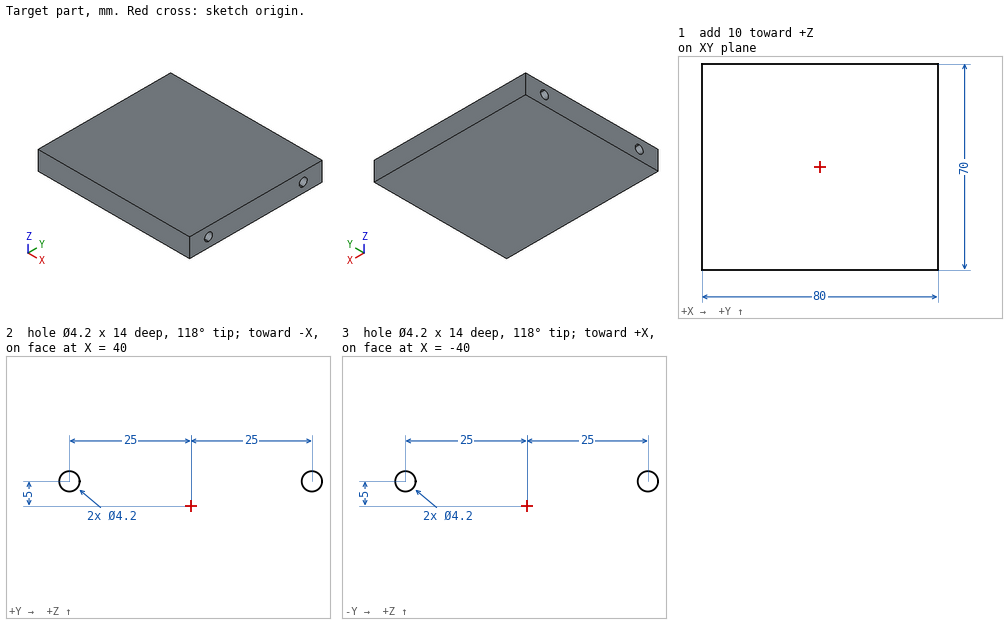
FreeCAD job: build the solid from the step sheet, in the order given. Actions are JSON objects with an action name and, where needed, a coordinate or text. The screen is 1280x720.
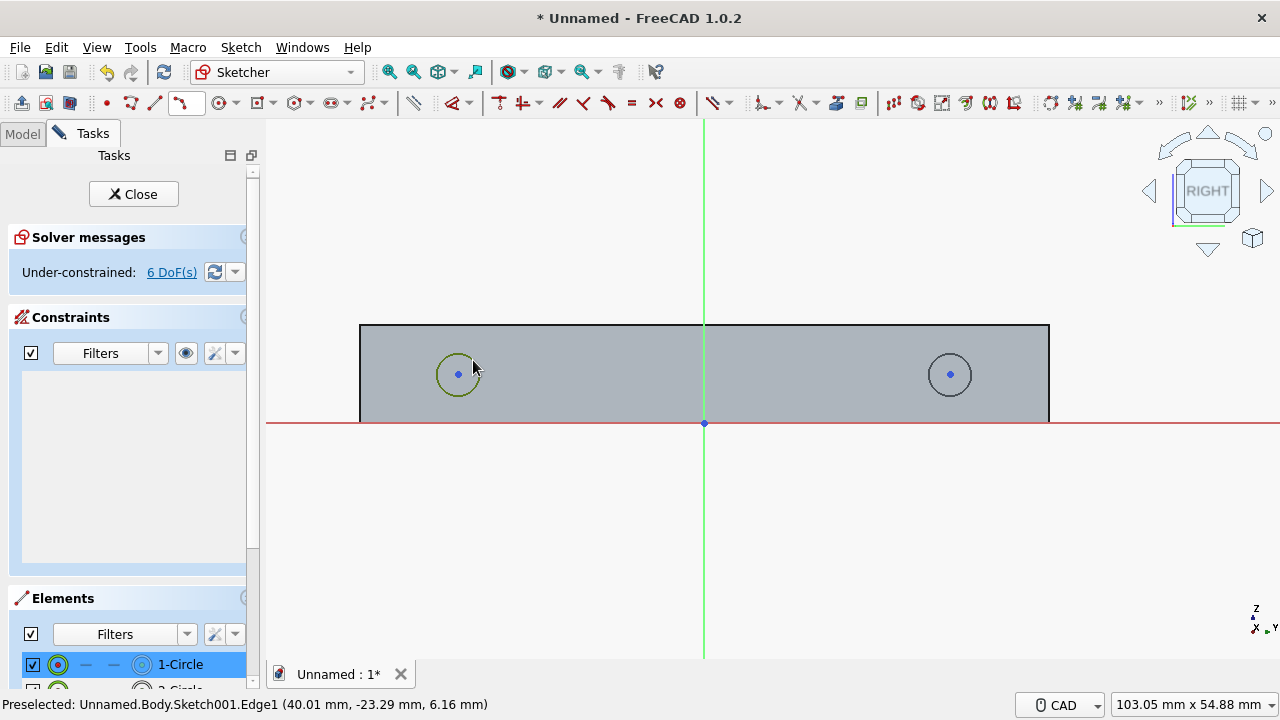
{"action": "left_click", "coordinate": [965, 360]}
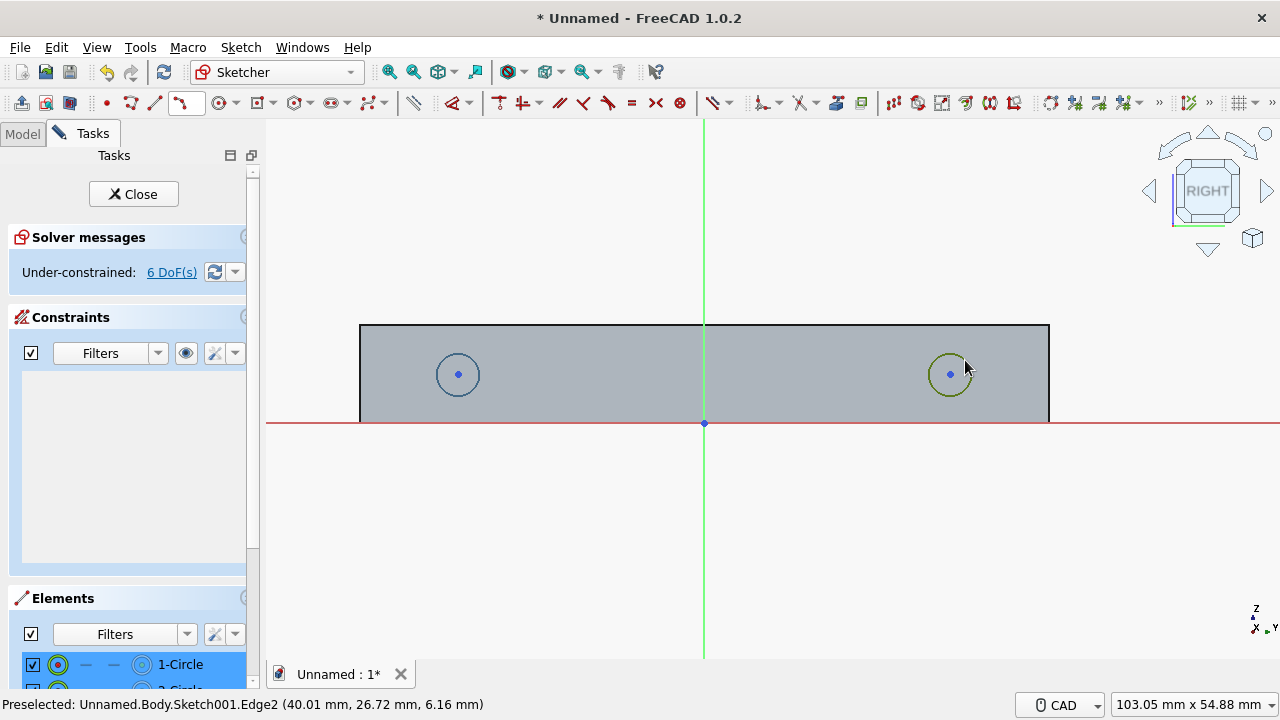
{"action": "left_click", "coordinate": [632, 104]}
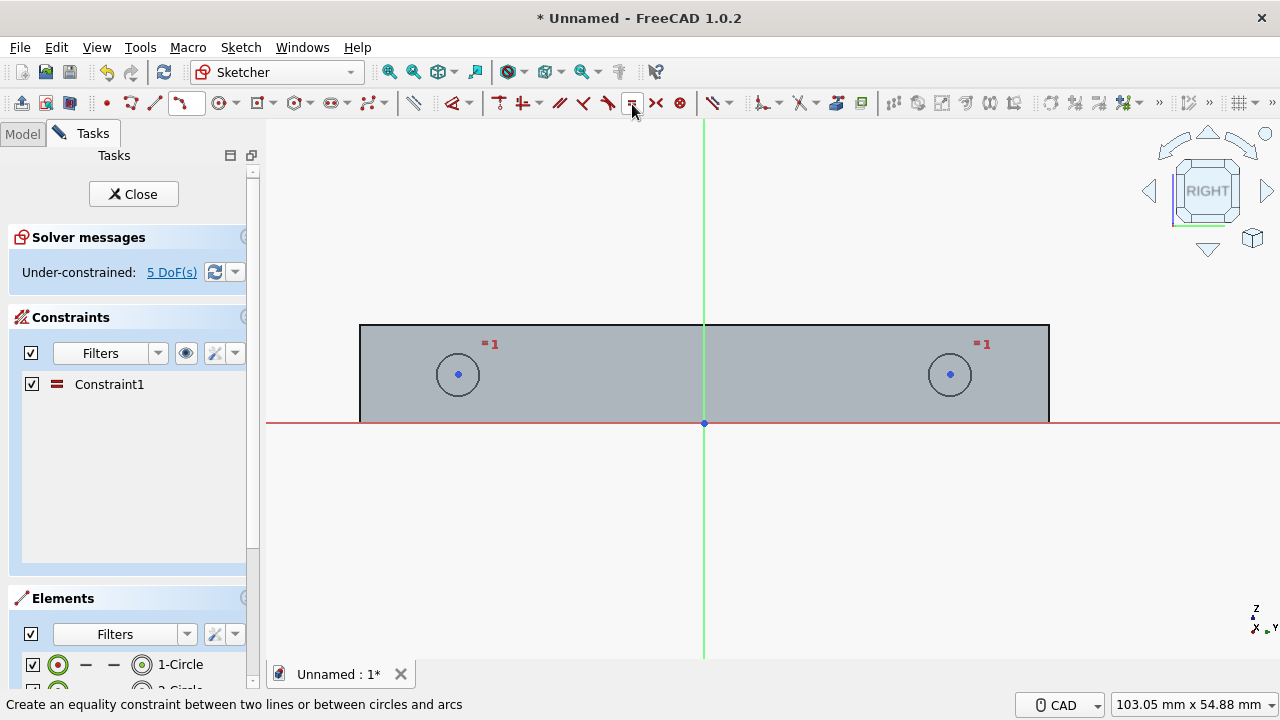
{"action": "left_click", "coordinate": [458, 375]}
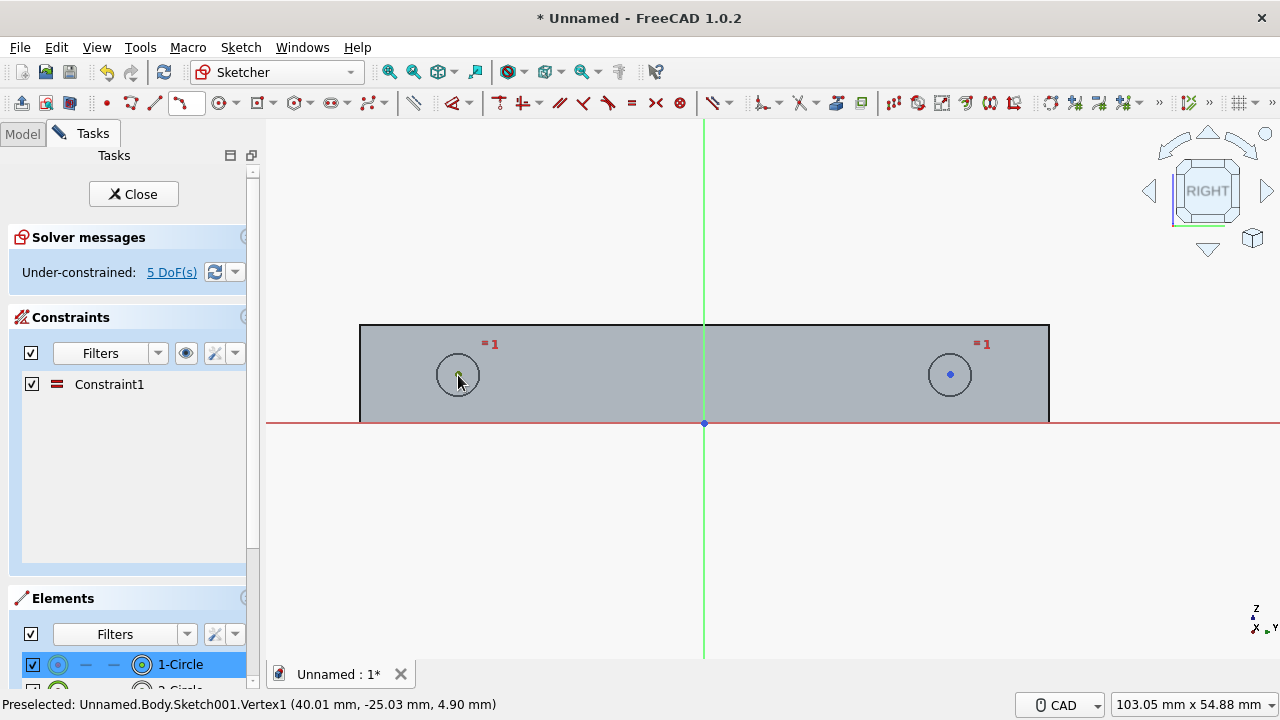
{"action": "left_click", "coordinate": [950, 375]}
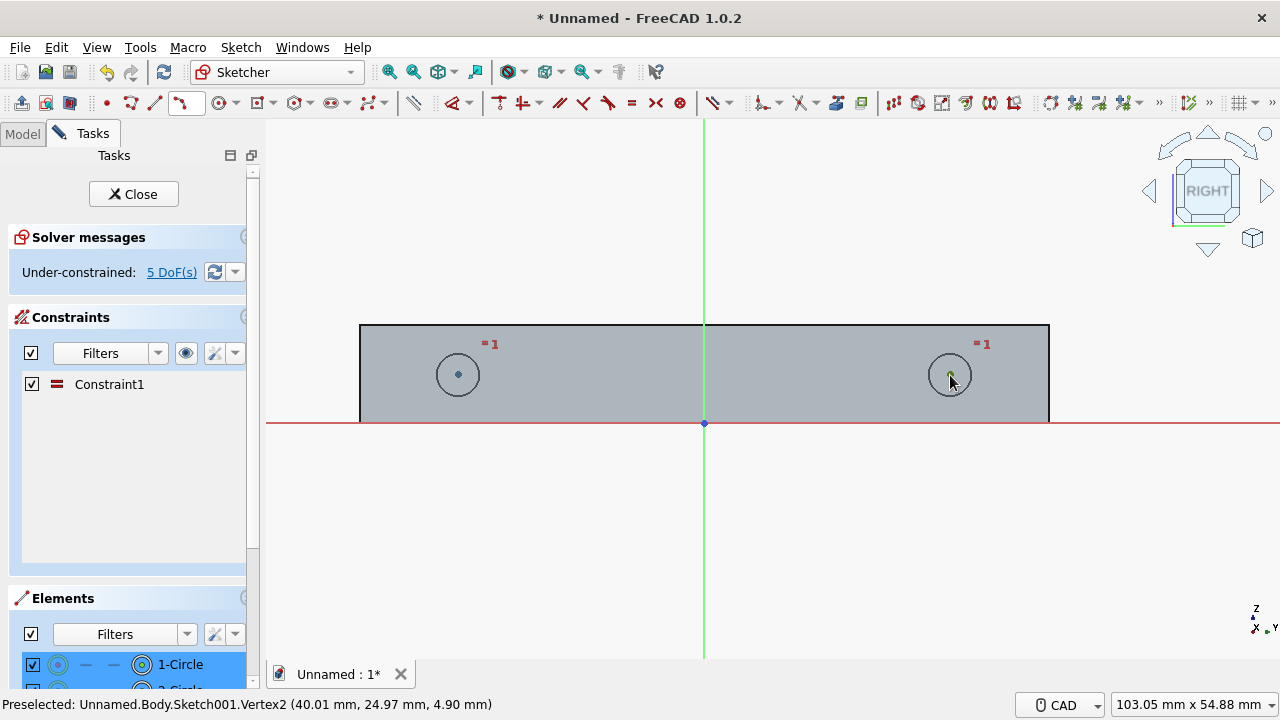
{"action": "key", "text": "h"}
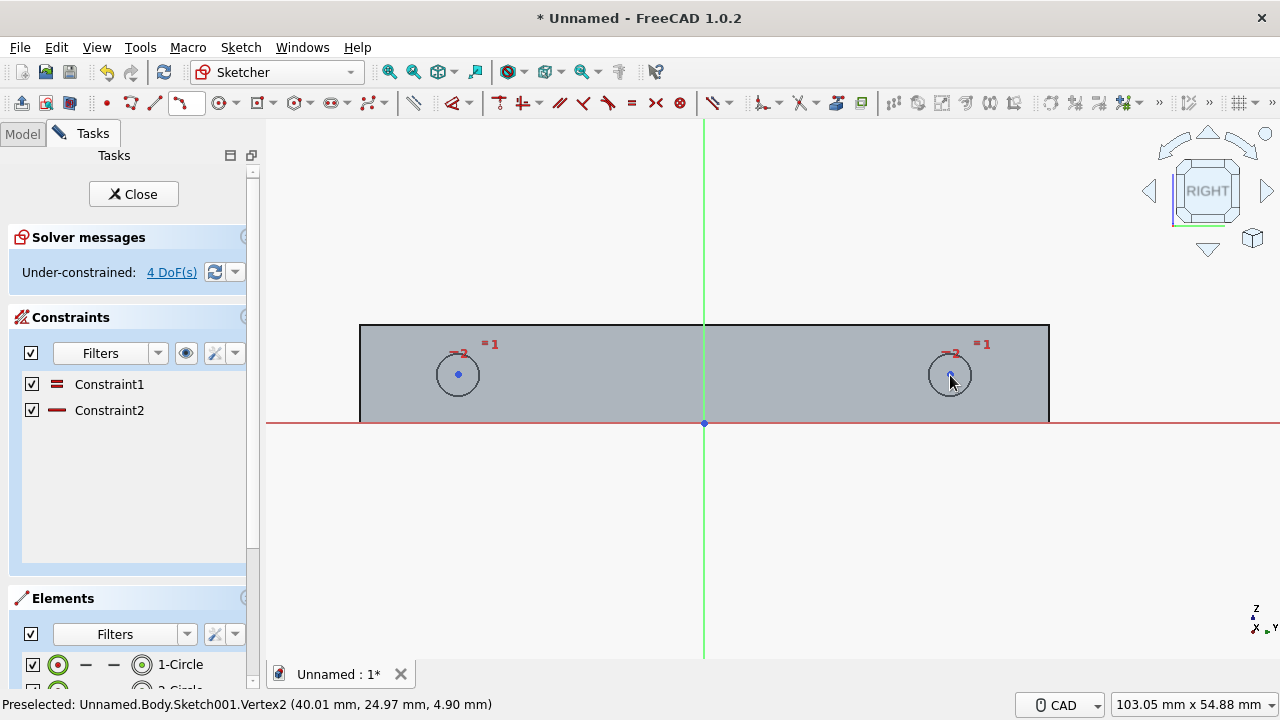
{"action": "left_click", "coordinate": [452, 104]}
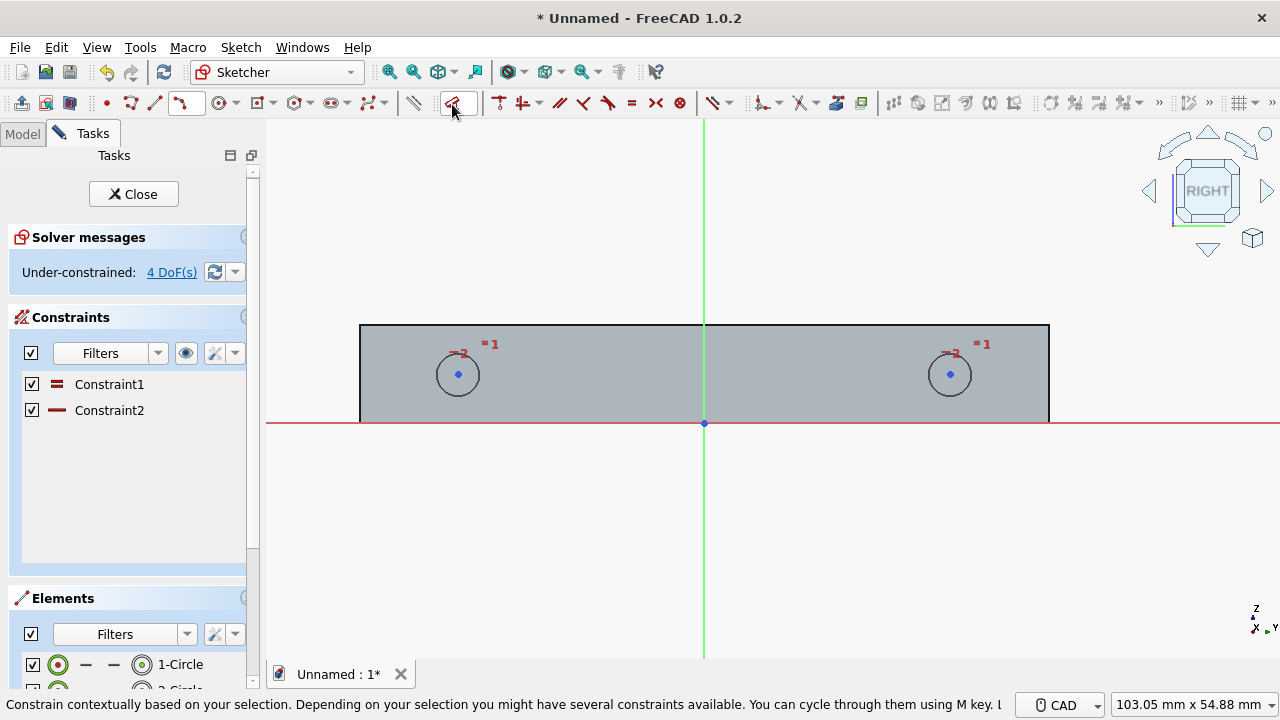
{"action": "left_click", "coordinate": [473, 360]}
{"action": "left_click", "coordinate": [496, 337]}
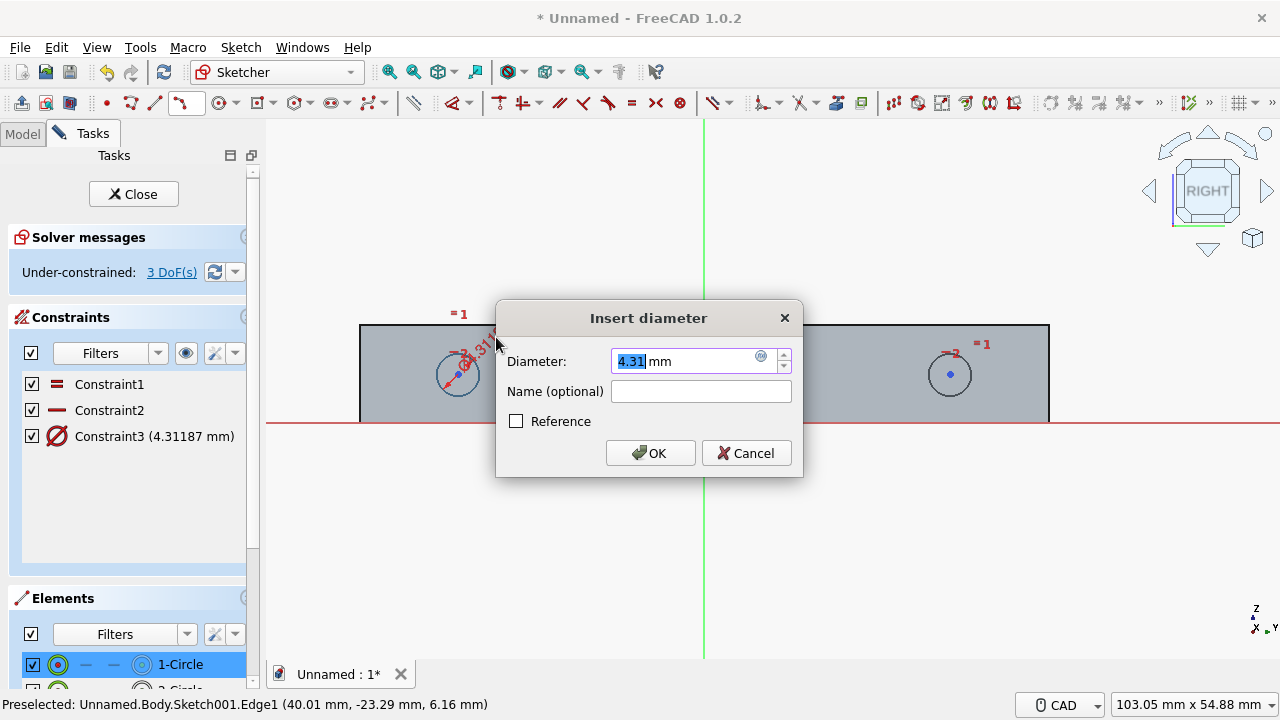
{"action": "type", "text": "4.2"}
{"action": "key", "text": "Return"}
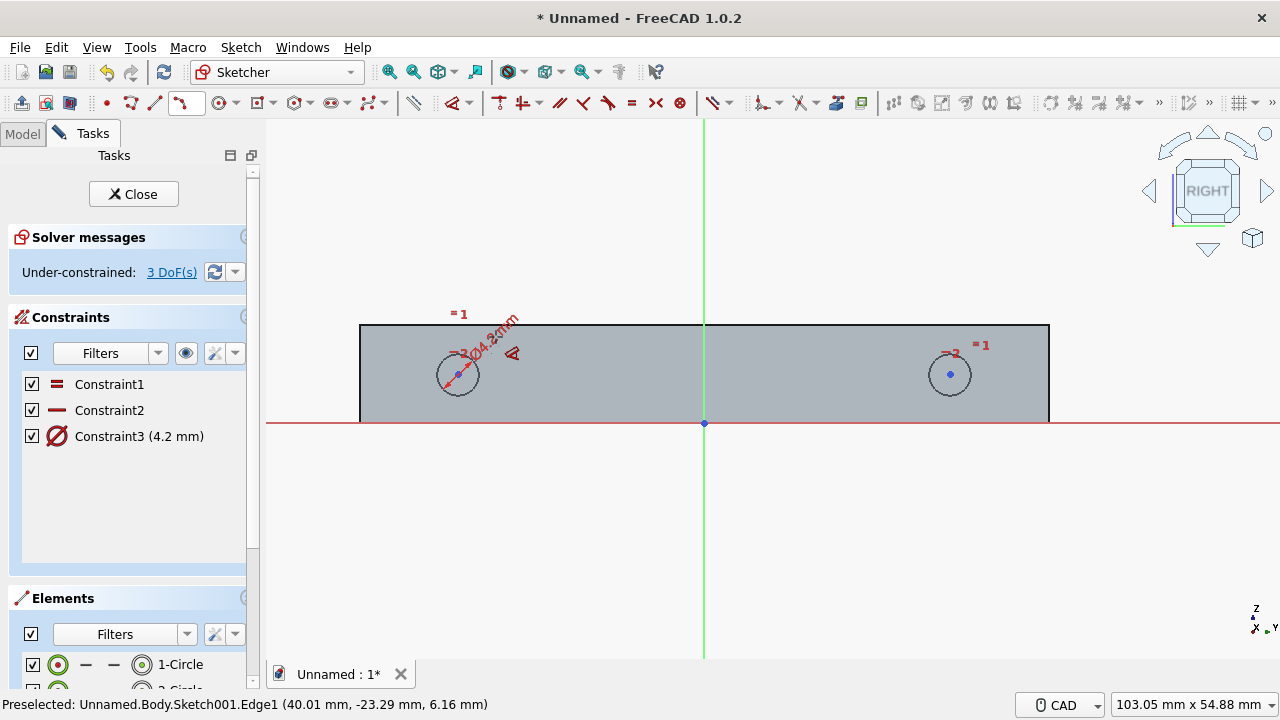
{"action": "left_click", "coordinate": [458, 375]}
{"action": "left_click", "coordinate": [424, 399]}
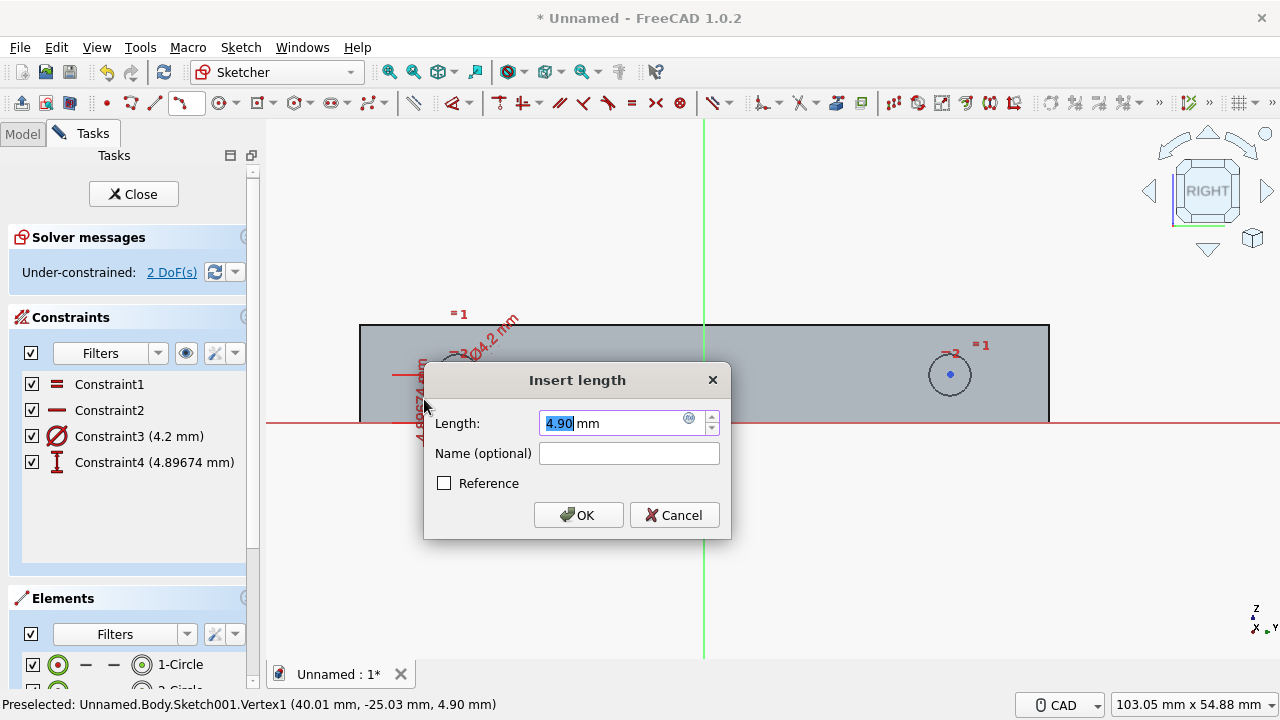
{"action": "type", "text": "5"}
{"action": "key", "text": "Return"}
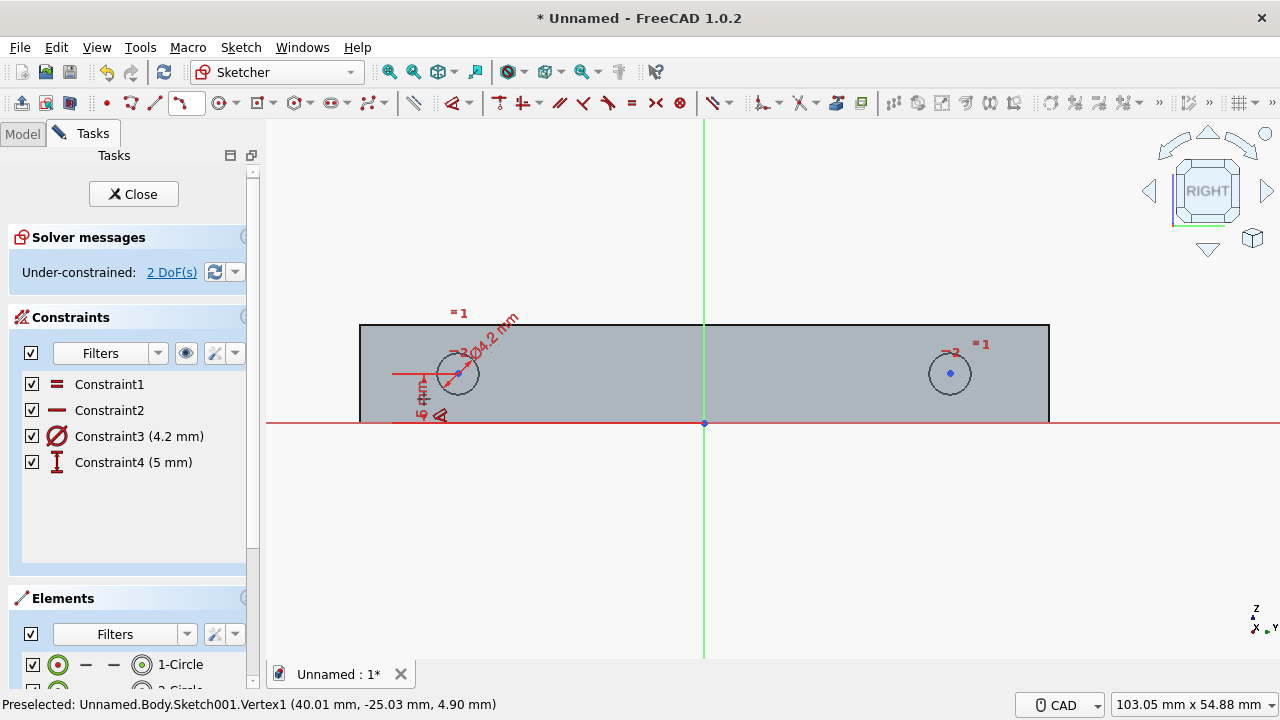
{"action": "left_click", "coordinate": [458, 374]}
{"action": "left_click", "coordinate": [581, 457]}